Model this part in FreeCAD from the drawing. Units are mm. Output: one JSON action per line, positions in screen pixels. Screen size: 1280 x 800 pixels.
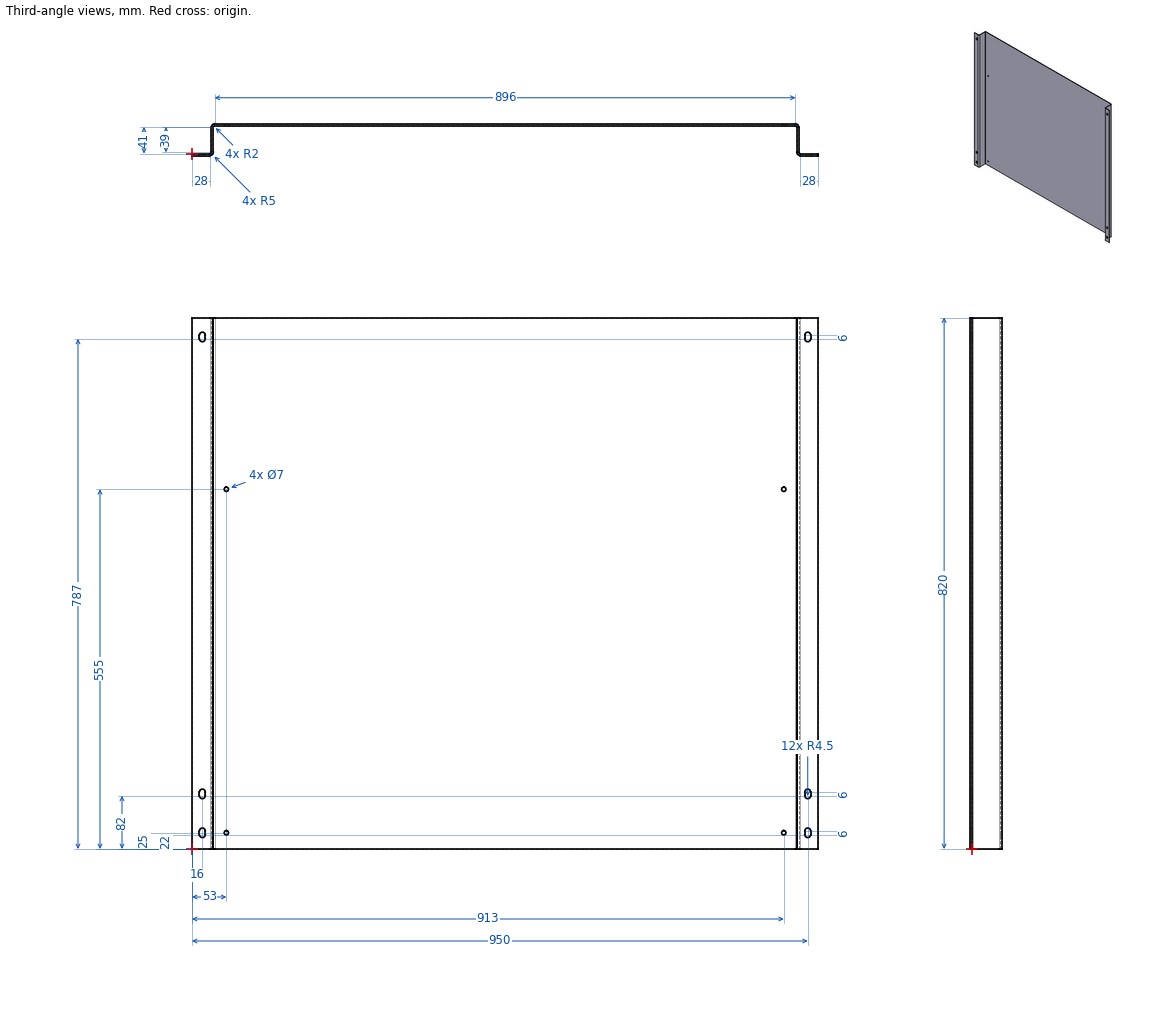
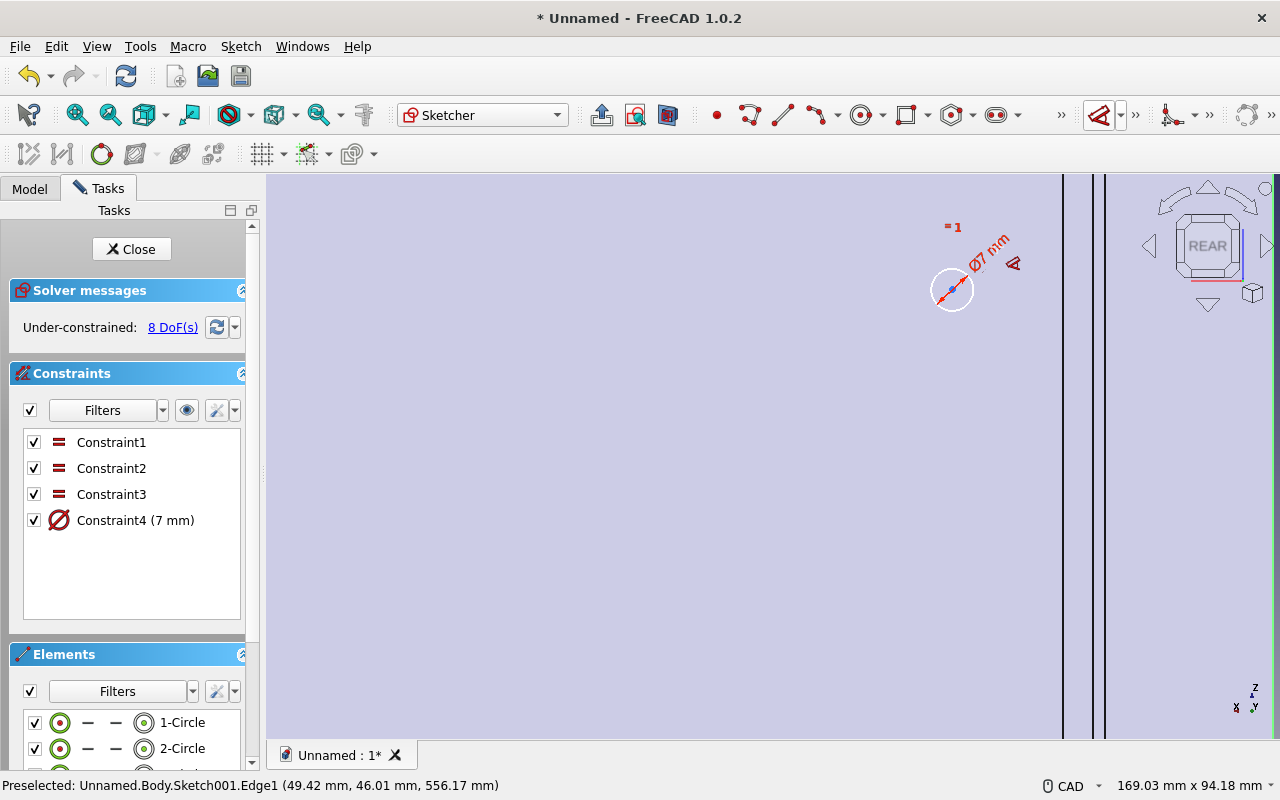
{"action": "scroll", "coordinate": [976, 272], "scroll_direction": "down", "scroll_amount": 11}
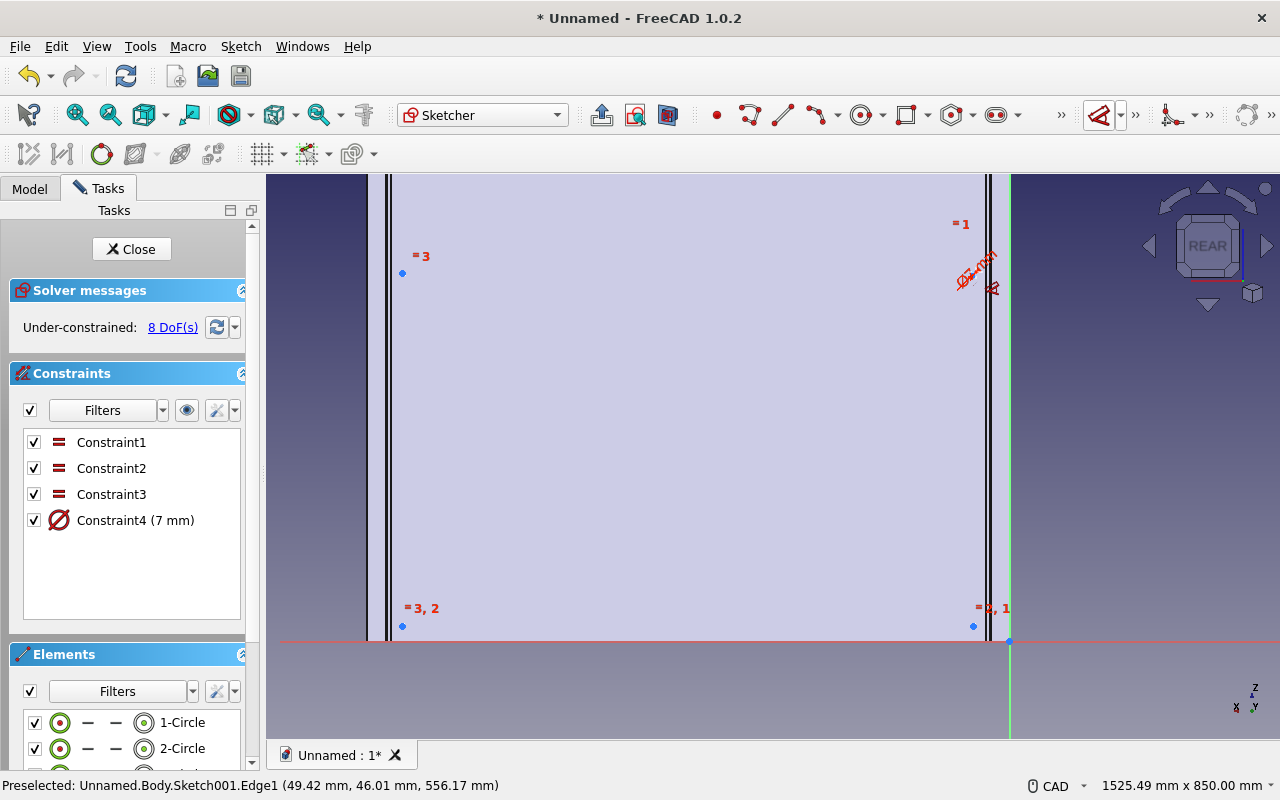
{"action": "left_click", "coordinate": [974, 274]}
{"action": "left_click", "coordinate": [992, 676]}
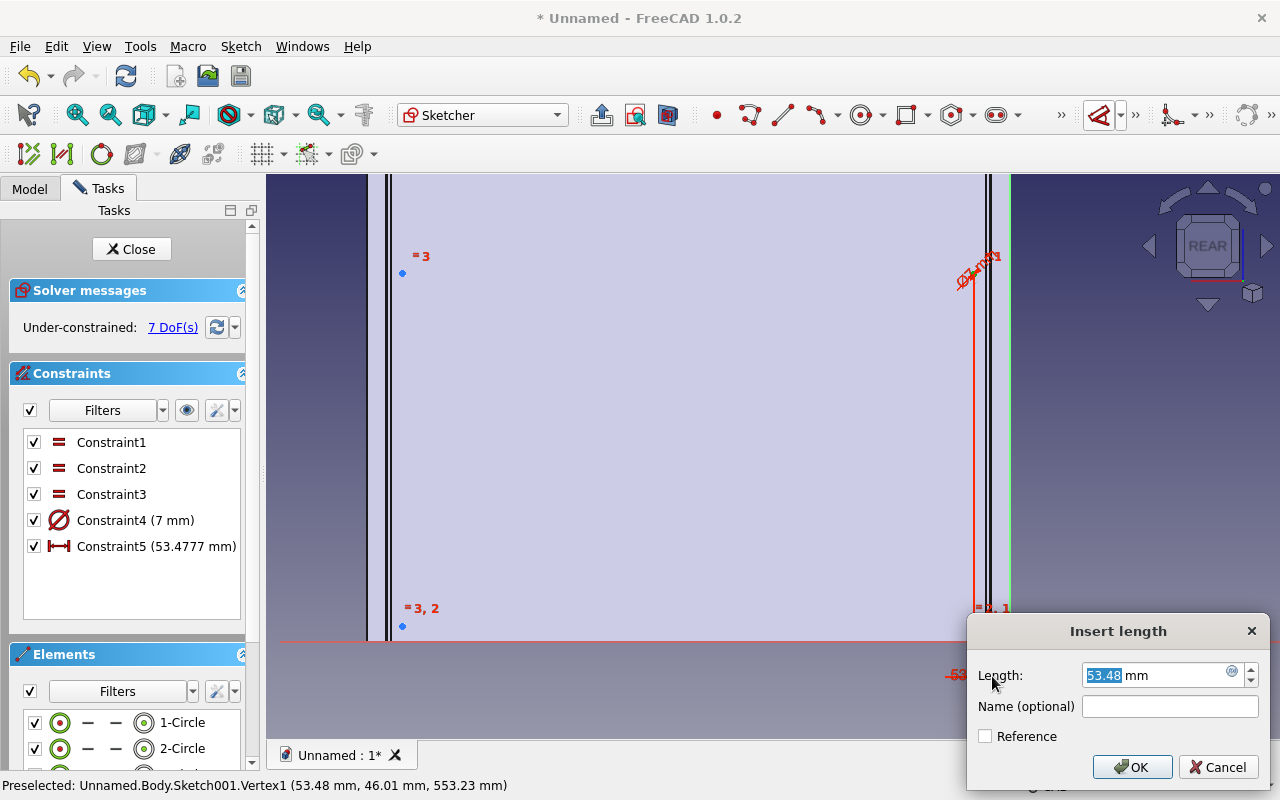
{"action": "type", "text": "53"}
{"action": "key", "text": "Return"}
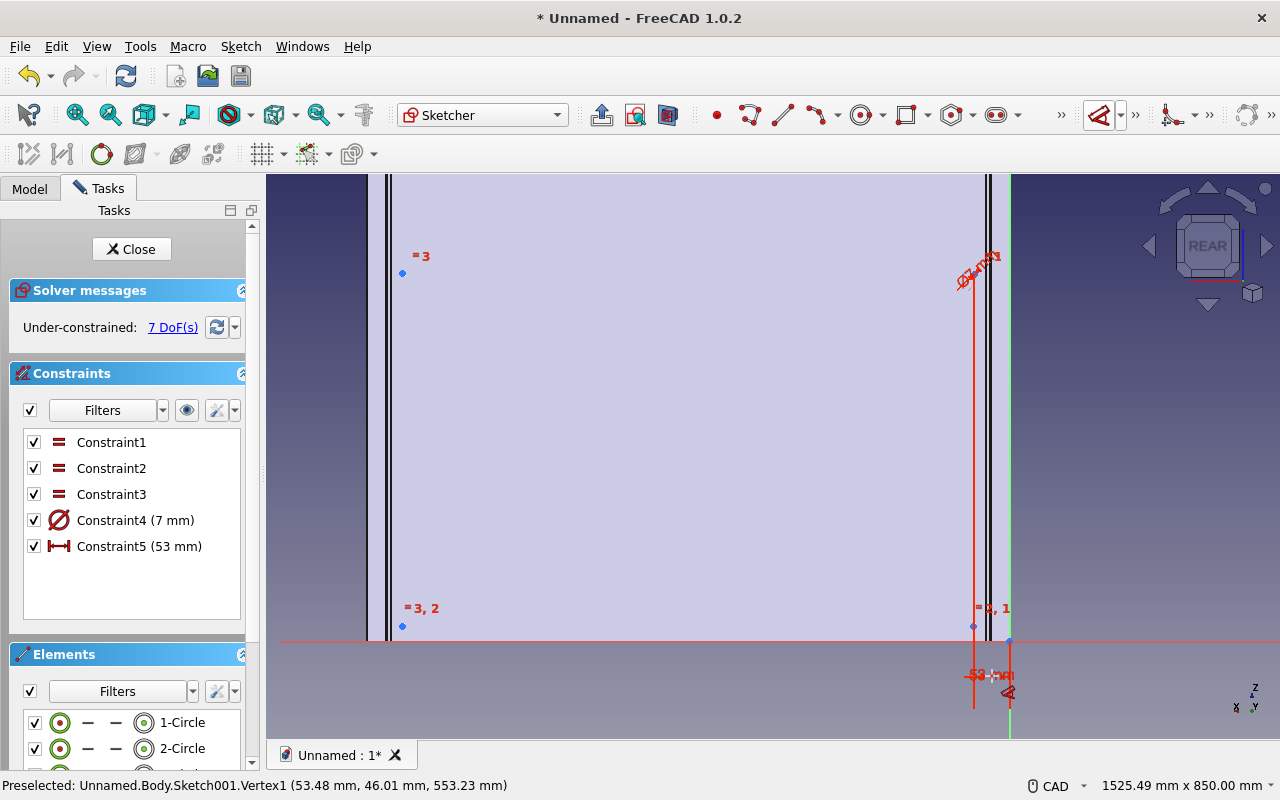
{"action": "left_click", "coordinate": [974, 626]}
{"action": "left_click", "coordinate": [992, 592]}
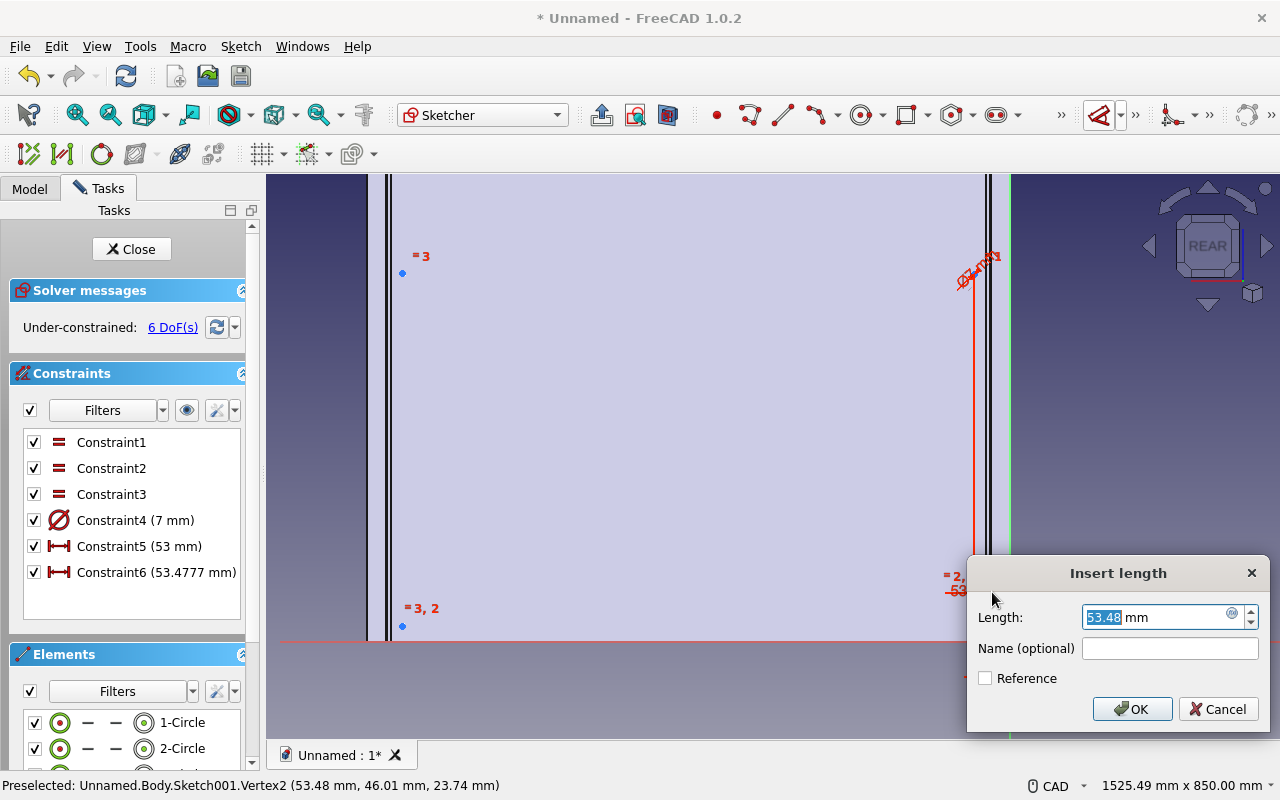
{"action": "type", "text": "53"}
{"action": "key", "text": "Return"}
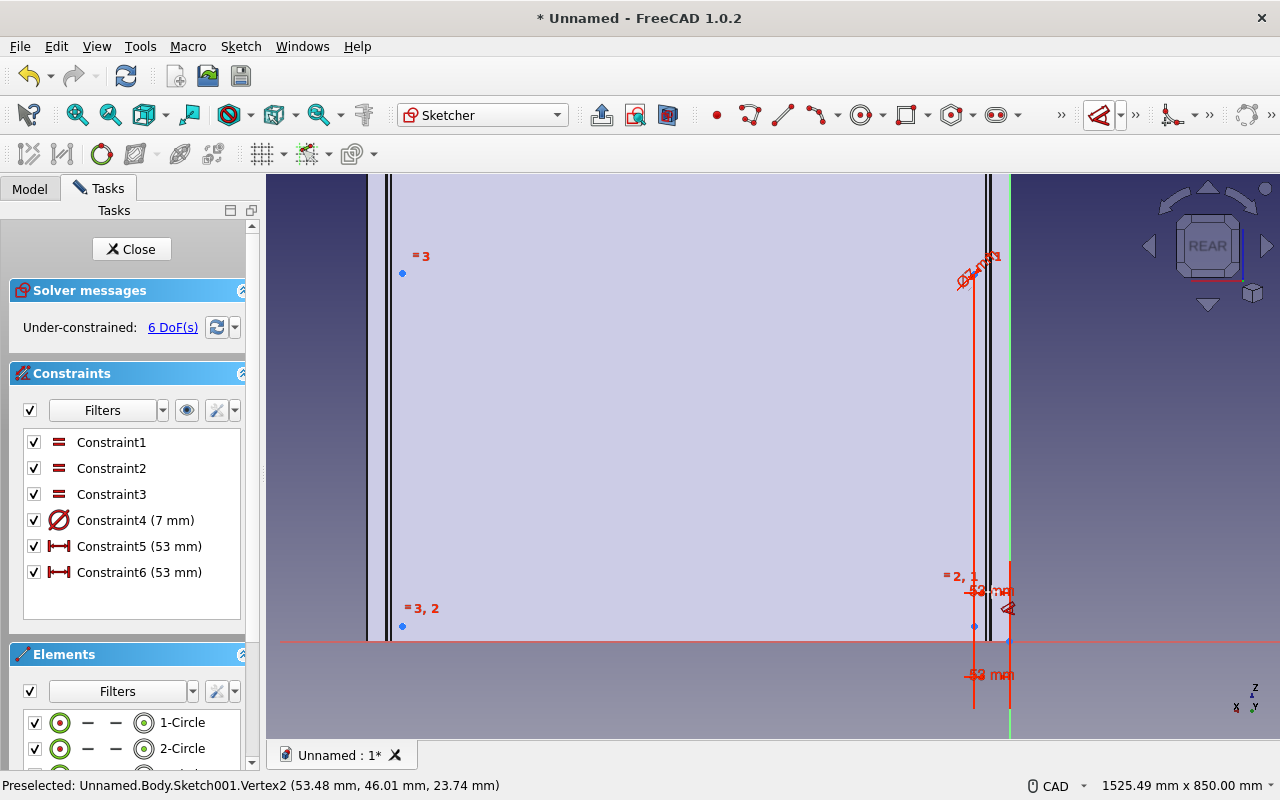
{"action": "scroll", "coordinate": [974, 626], "scroll_direction": "up", "scroll_amount": 5}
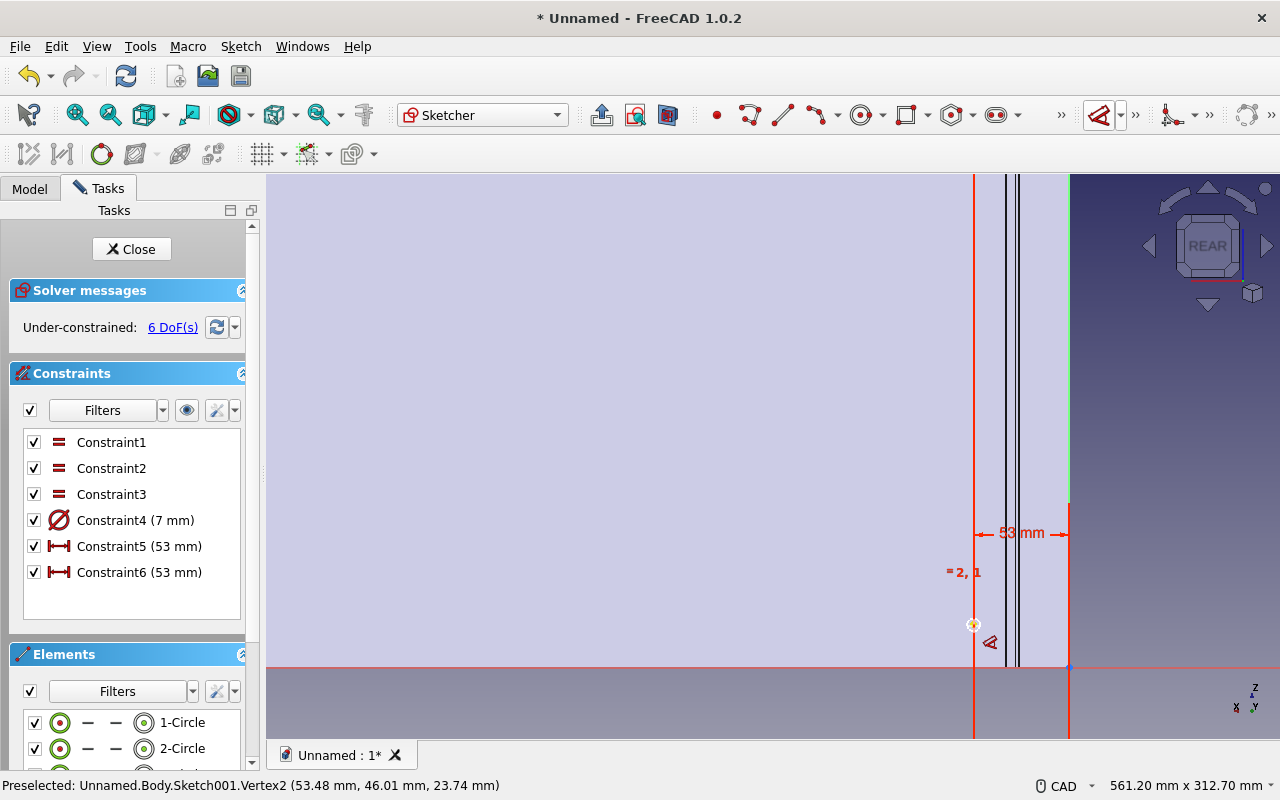
{"action": "left_click", "coordinate": [974, 625]}
{"action": "left_click", "coordinate": [1103, 646]}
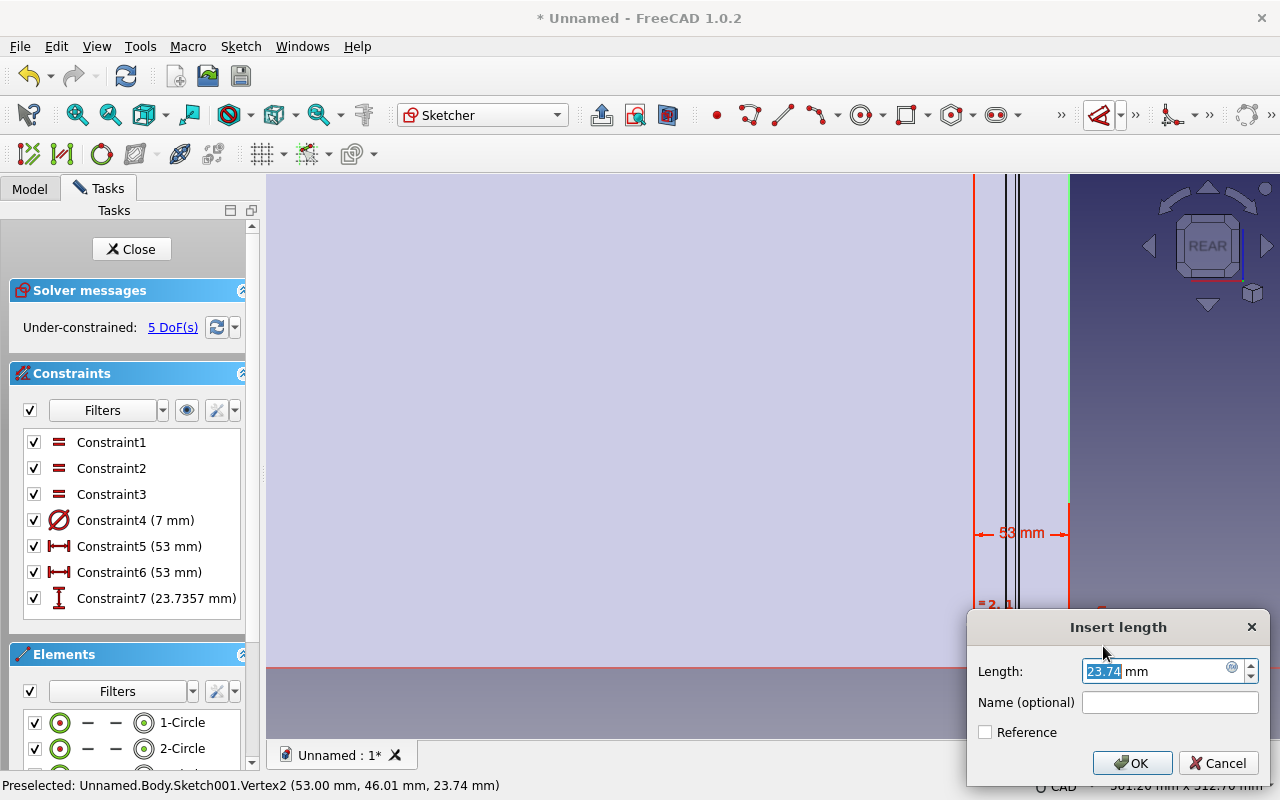
{"action": "type", "text": "25"}
{"action": "key", "text": "Return"}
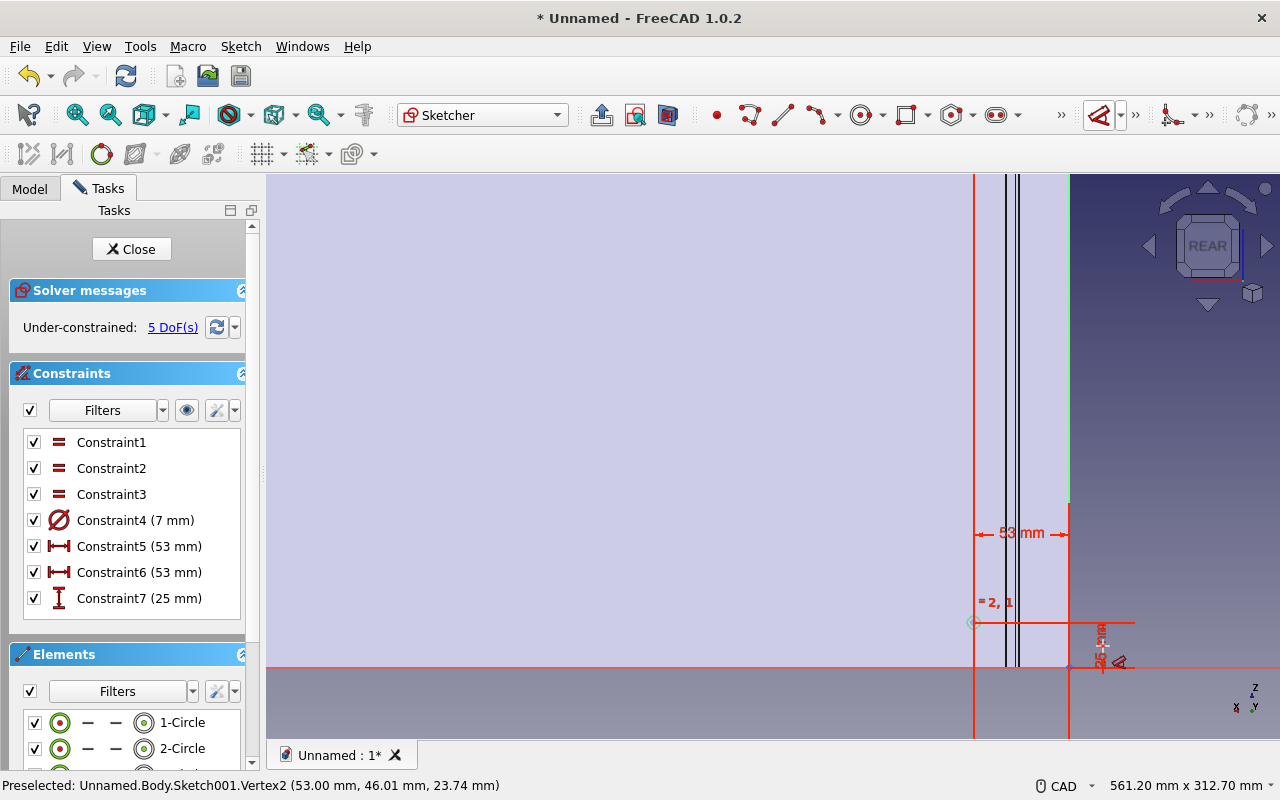
{"action": "scroll", "coordinate": [974, 627], "scroll_direction": "down", "scroll_amount": 5}